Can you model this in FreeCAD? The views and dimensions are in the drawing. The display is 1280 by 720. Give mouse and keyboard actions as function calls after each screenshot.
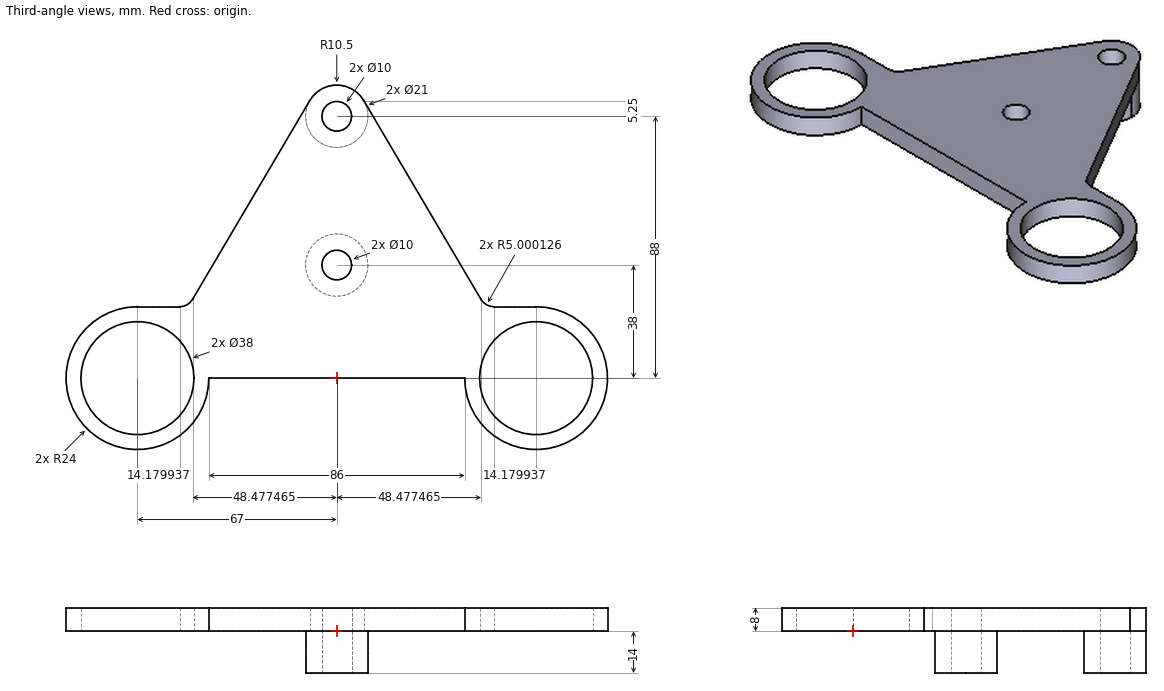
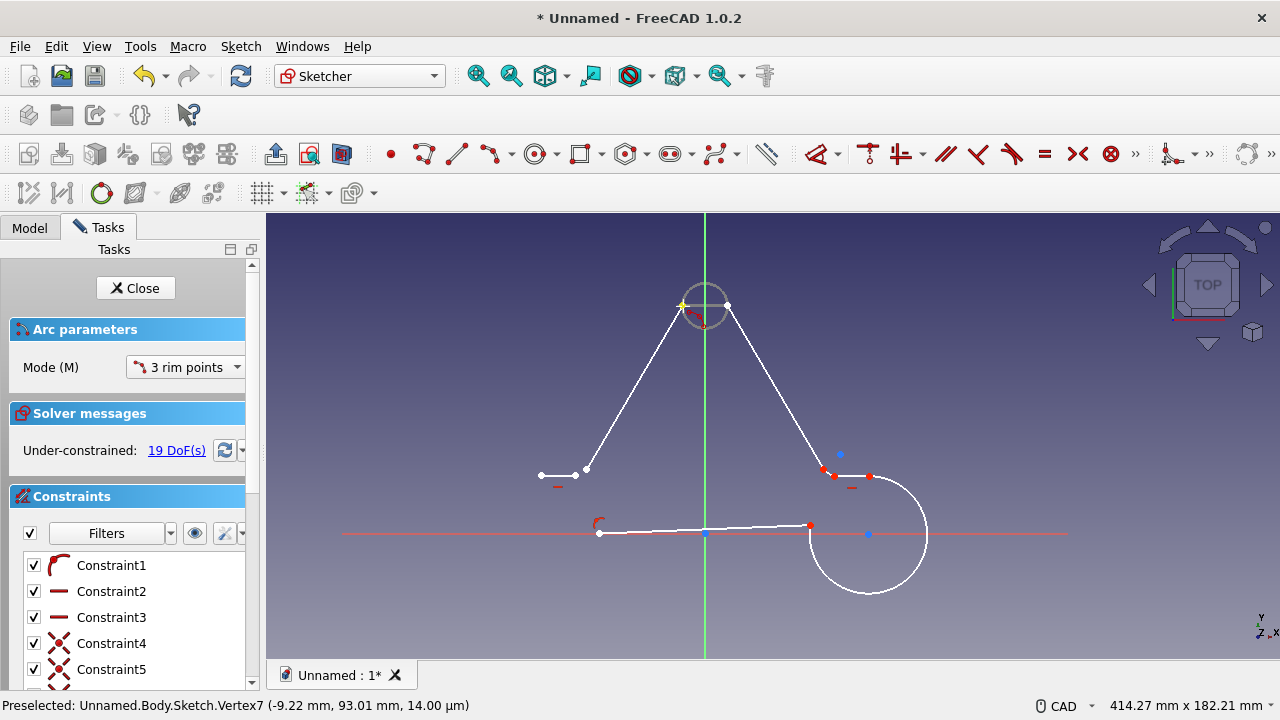
scroll(716, 295, up, 3)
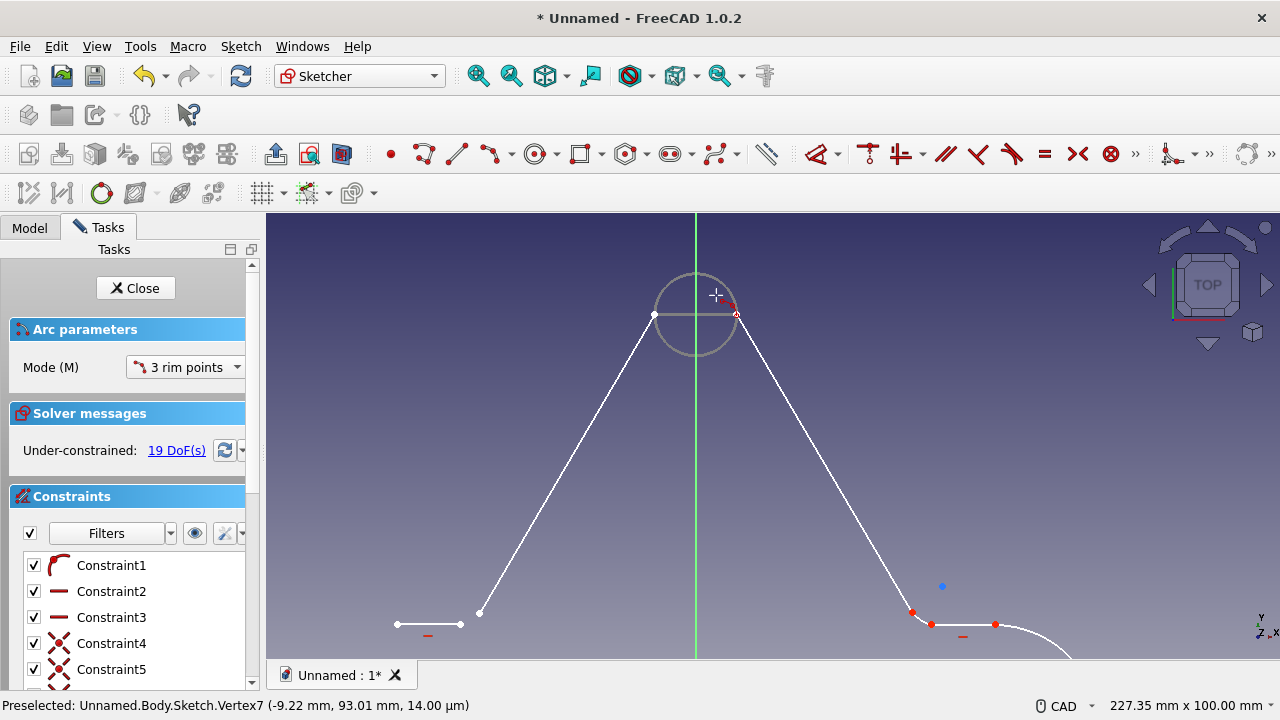
click(715, 294)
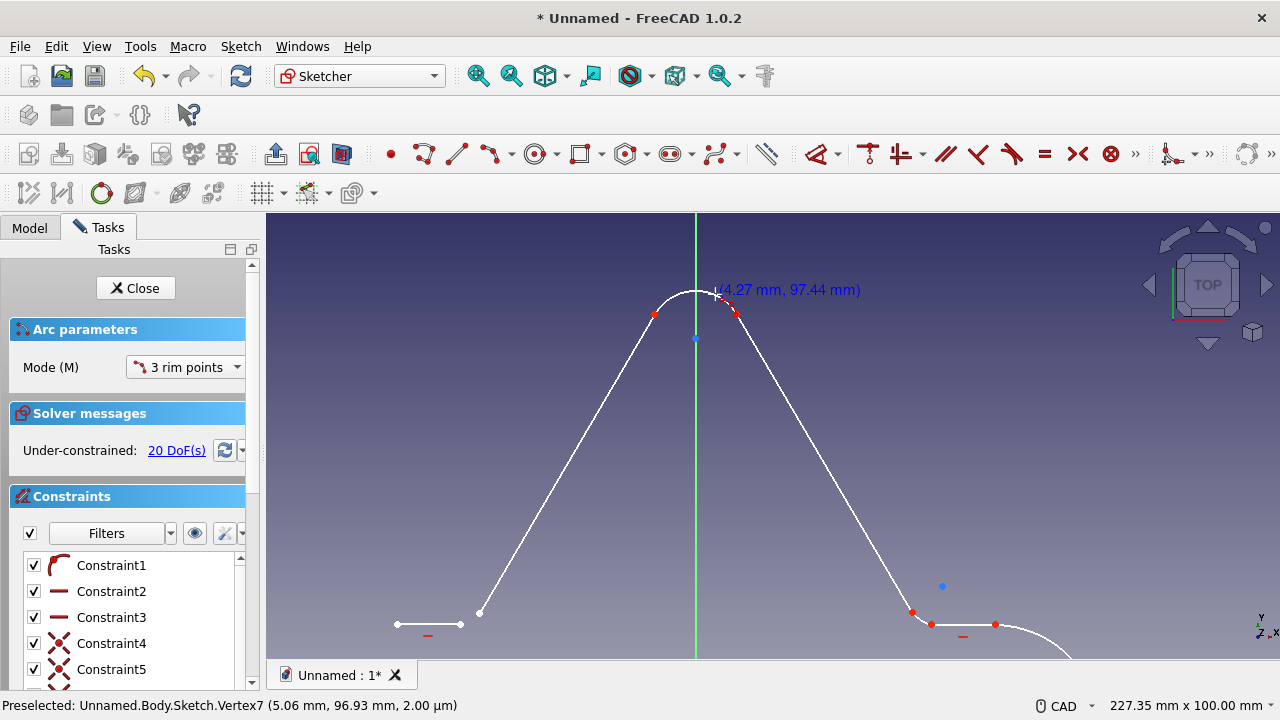
click(480, 614)
click(460, 624)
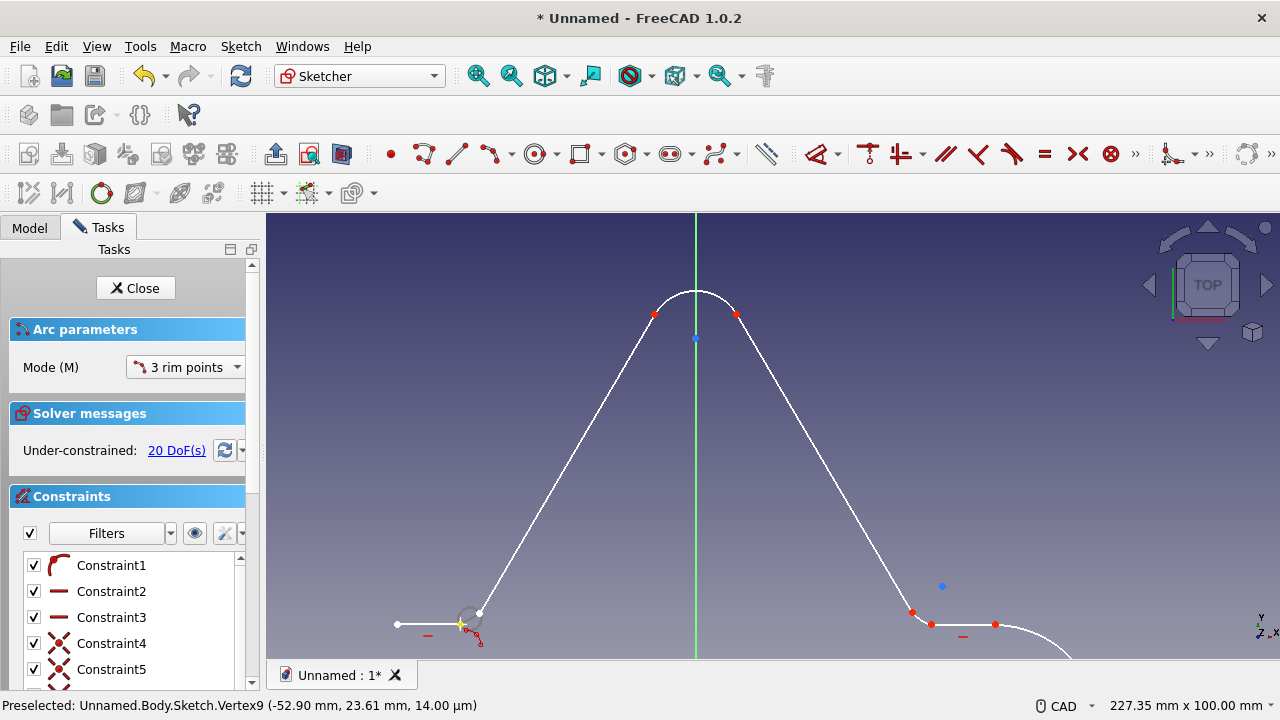
scroll(472, 620, up, 9)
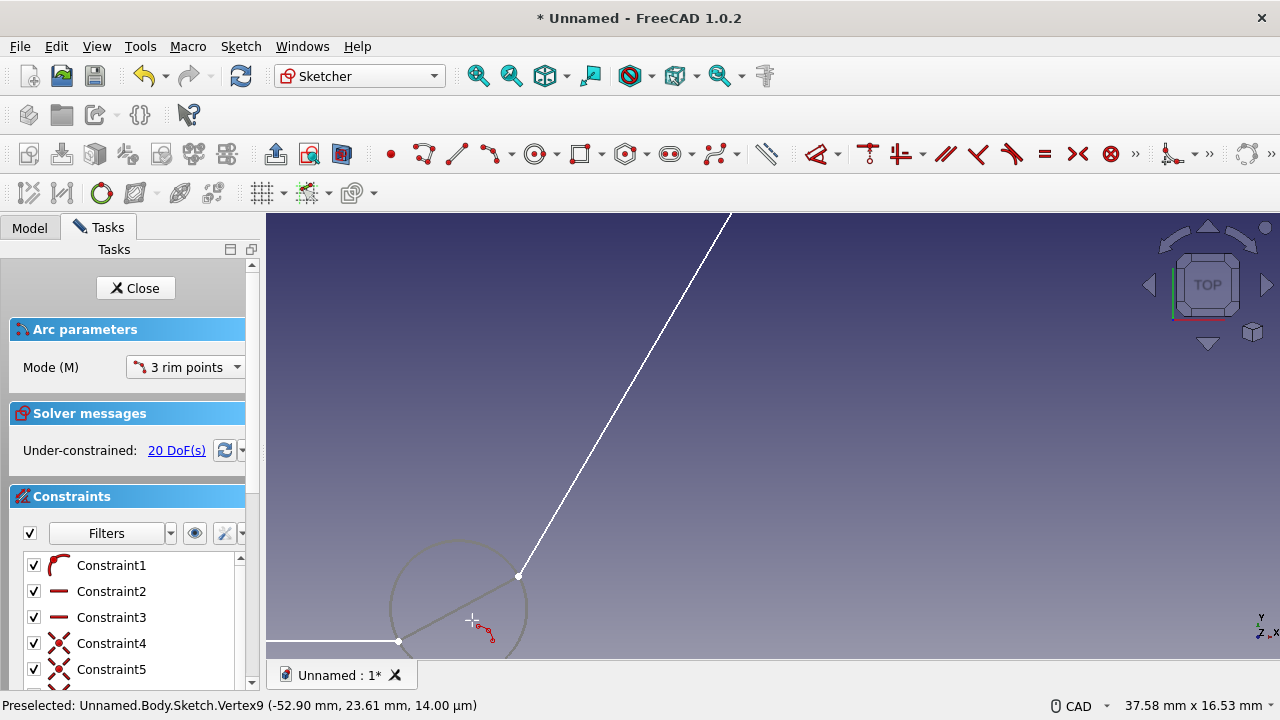
click(468, 613)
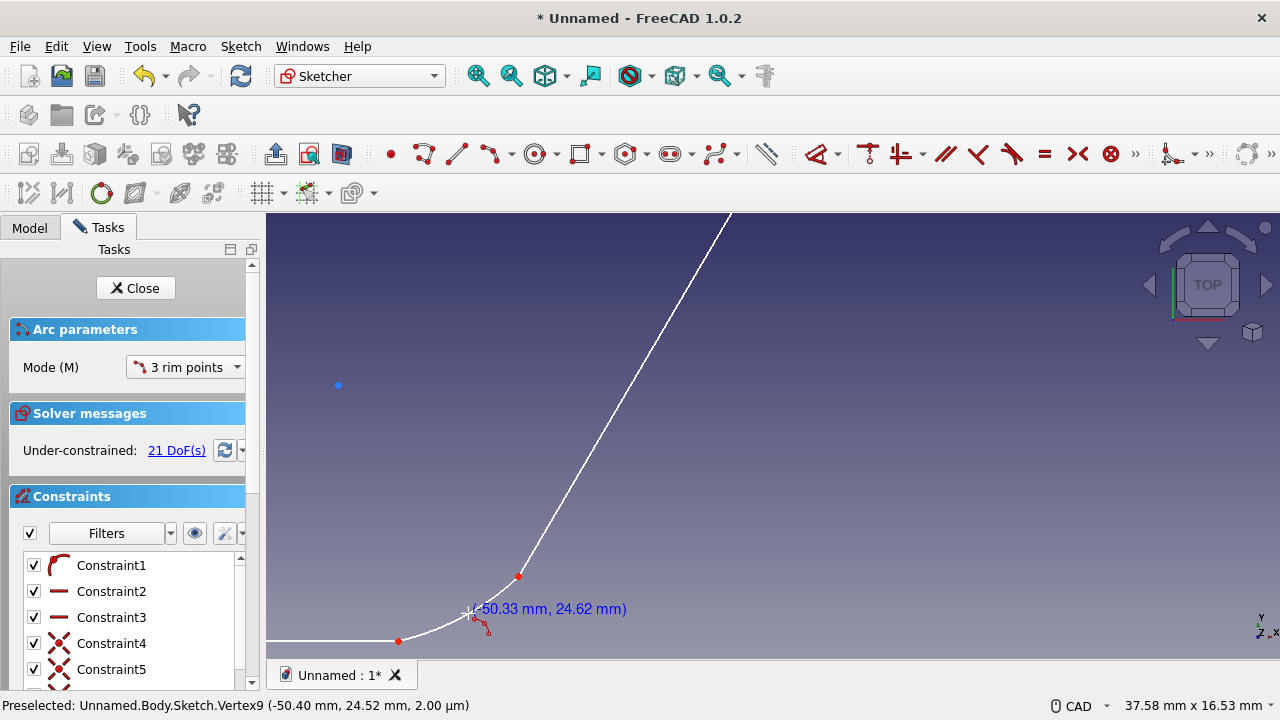
scroll(593, 459, down, 12)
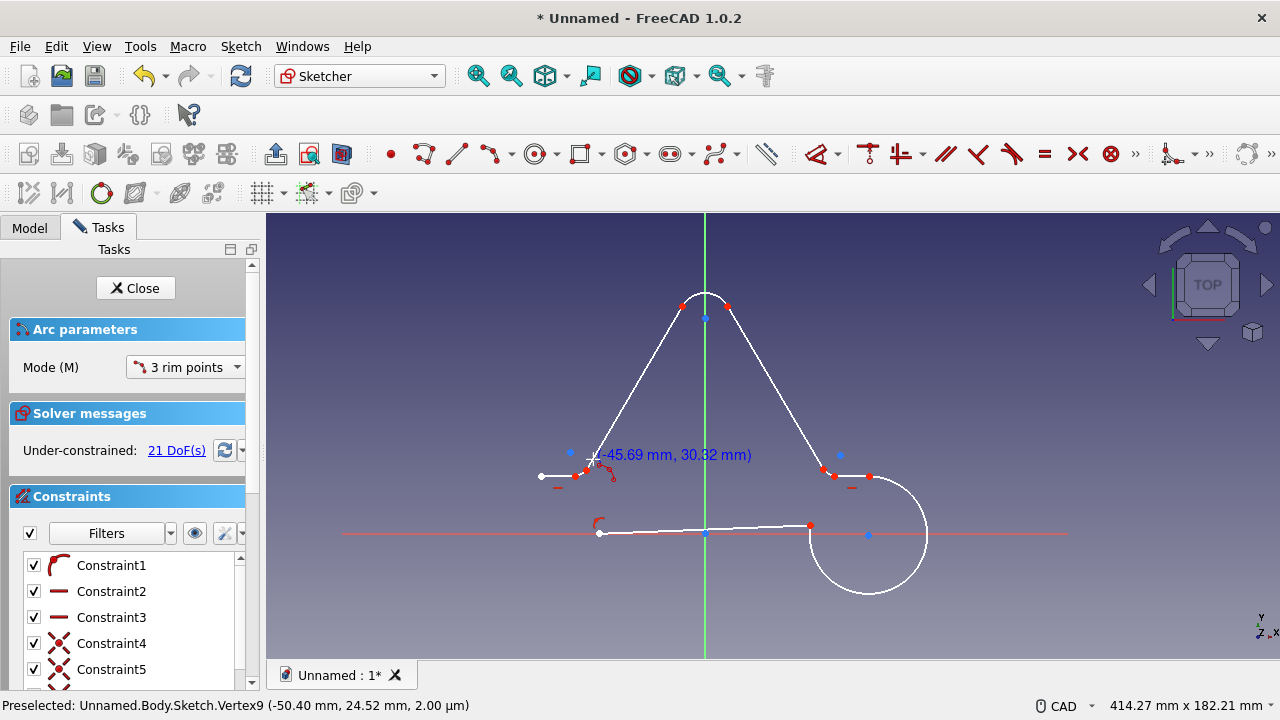
click(541, 476)
click(600, 534)
click(500, 575)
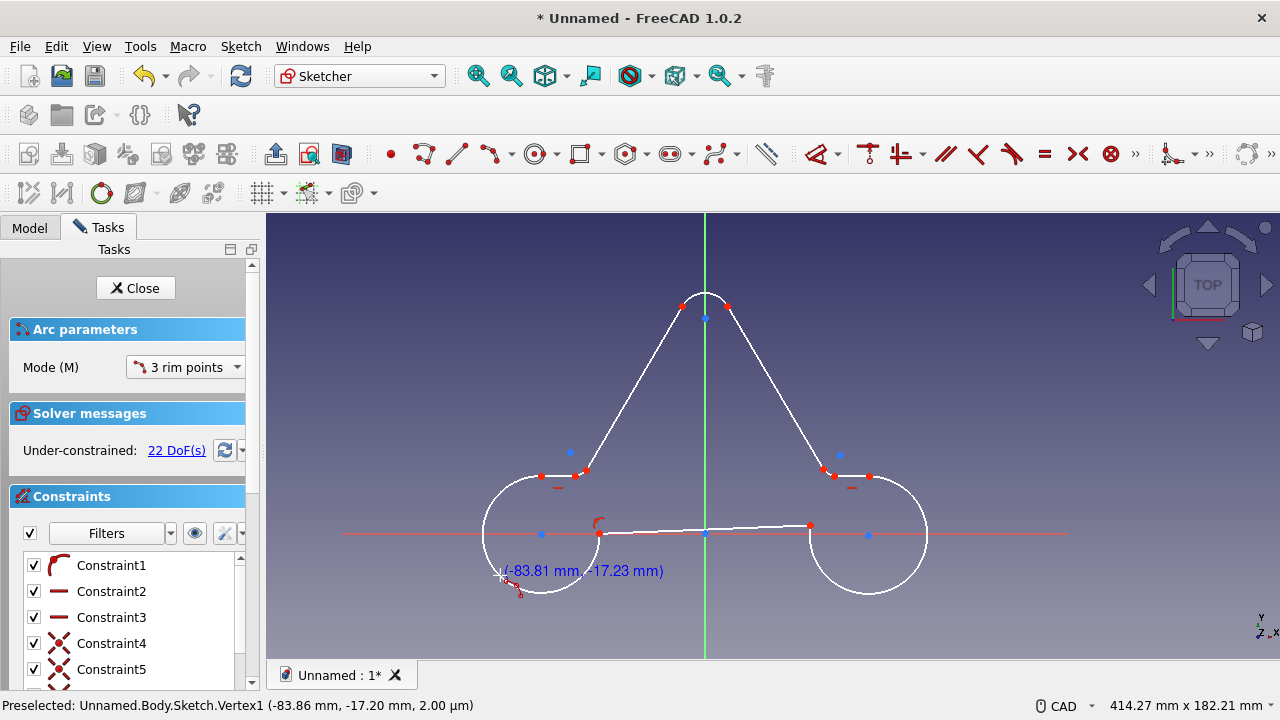
key(g)
key(c)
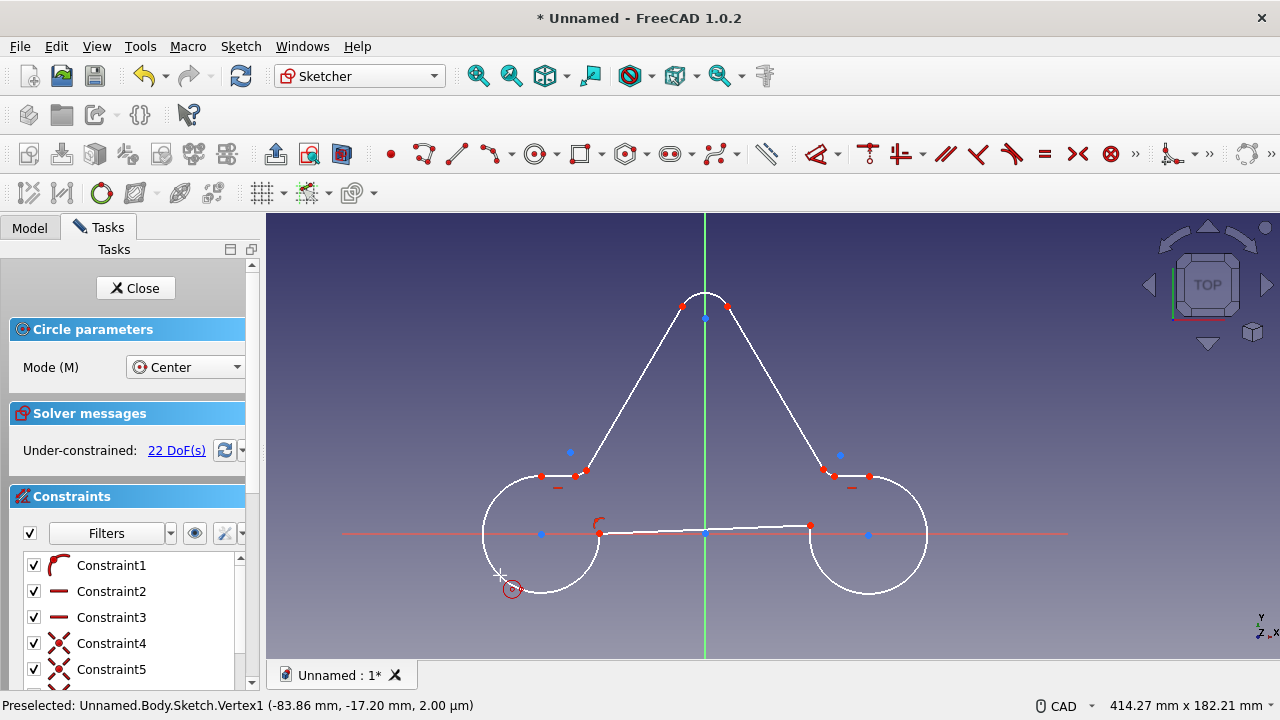
click(541, 534)
click(574, 501)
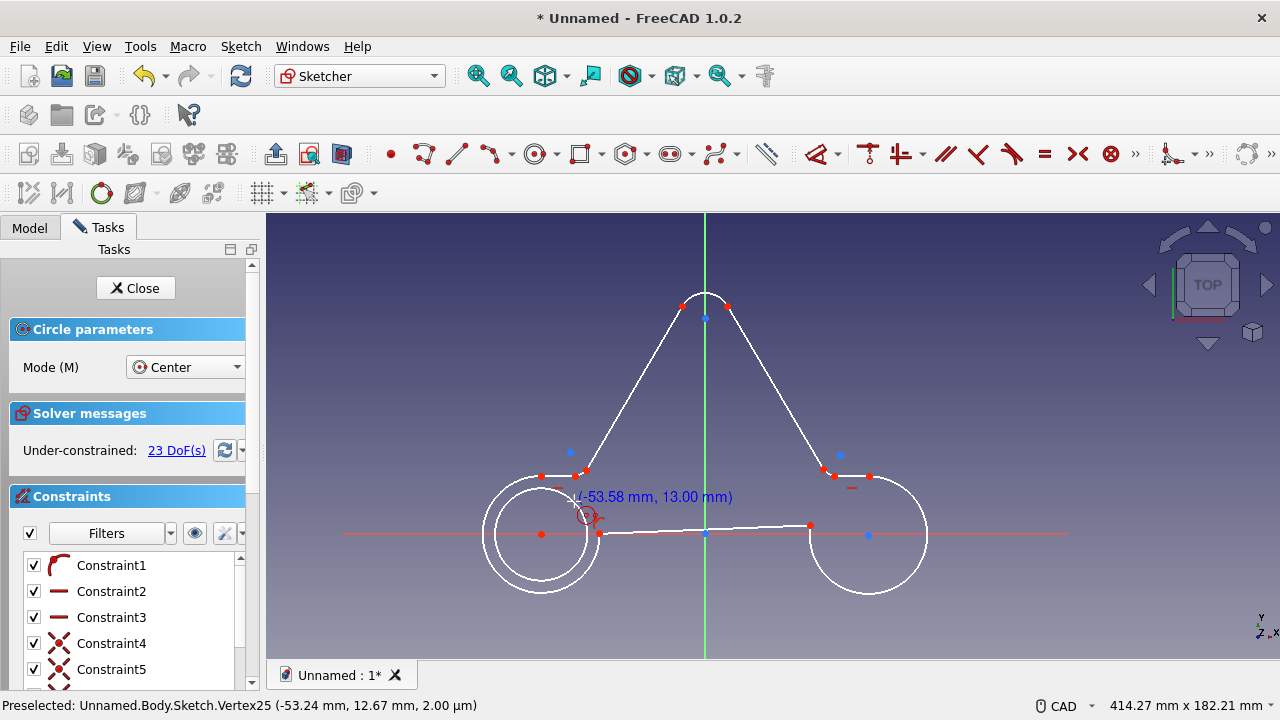
click(869, 534)
click(836, 501)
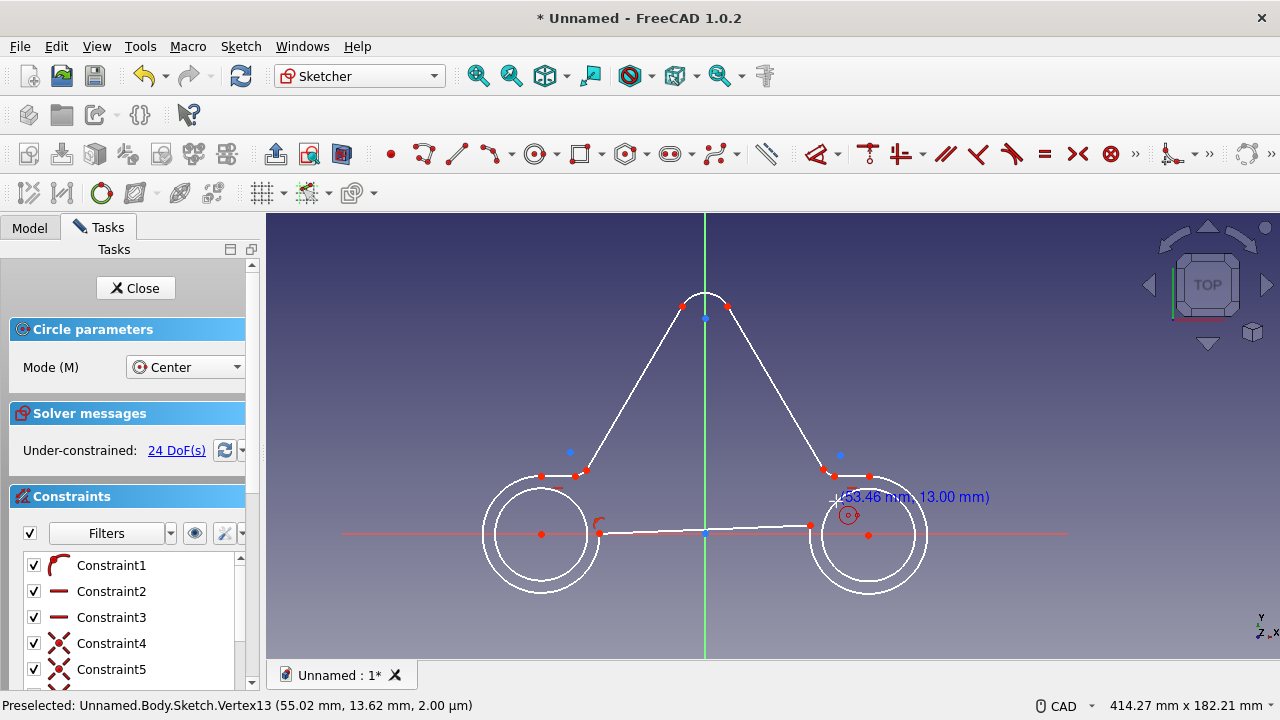
scroll(705, 441, up, 4)